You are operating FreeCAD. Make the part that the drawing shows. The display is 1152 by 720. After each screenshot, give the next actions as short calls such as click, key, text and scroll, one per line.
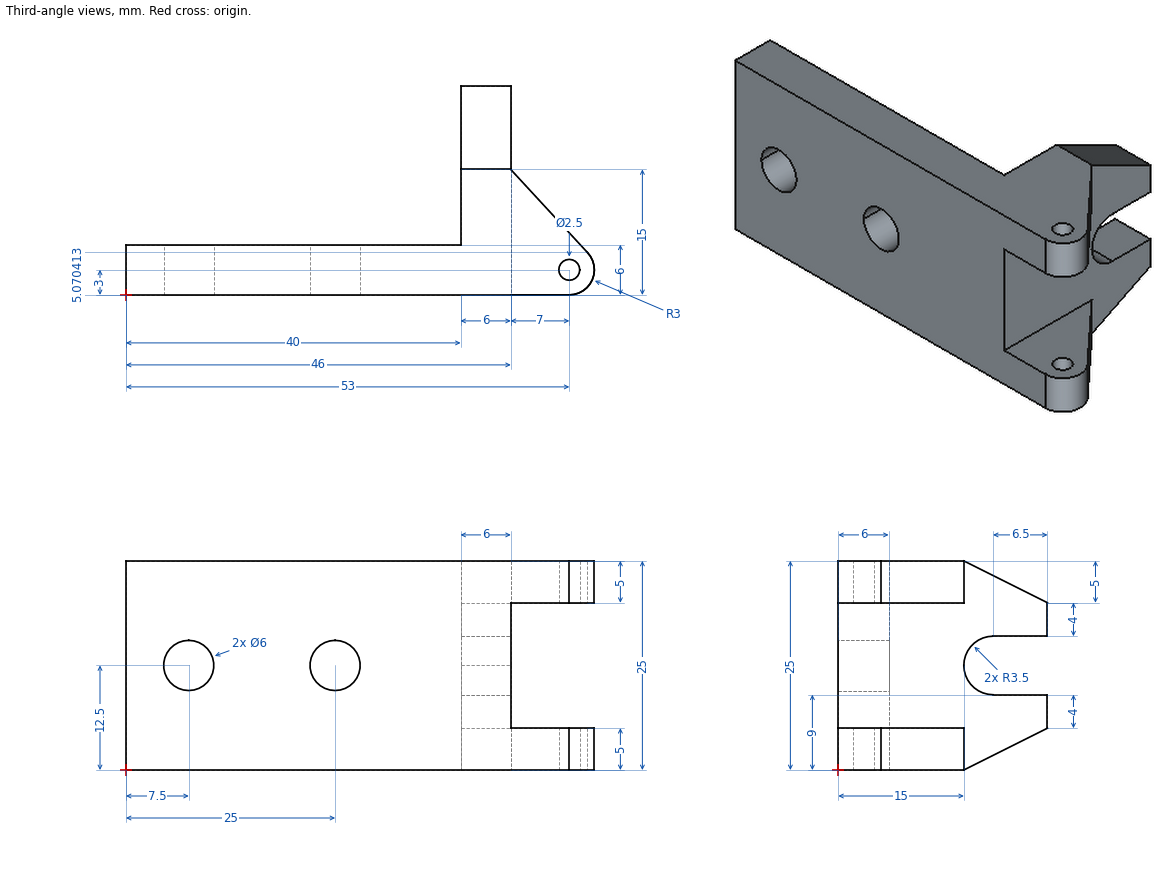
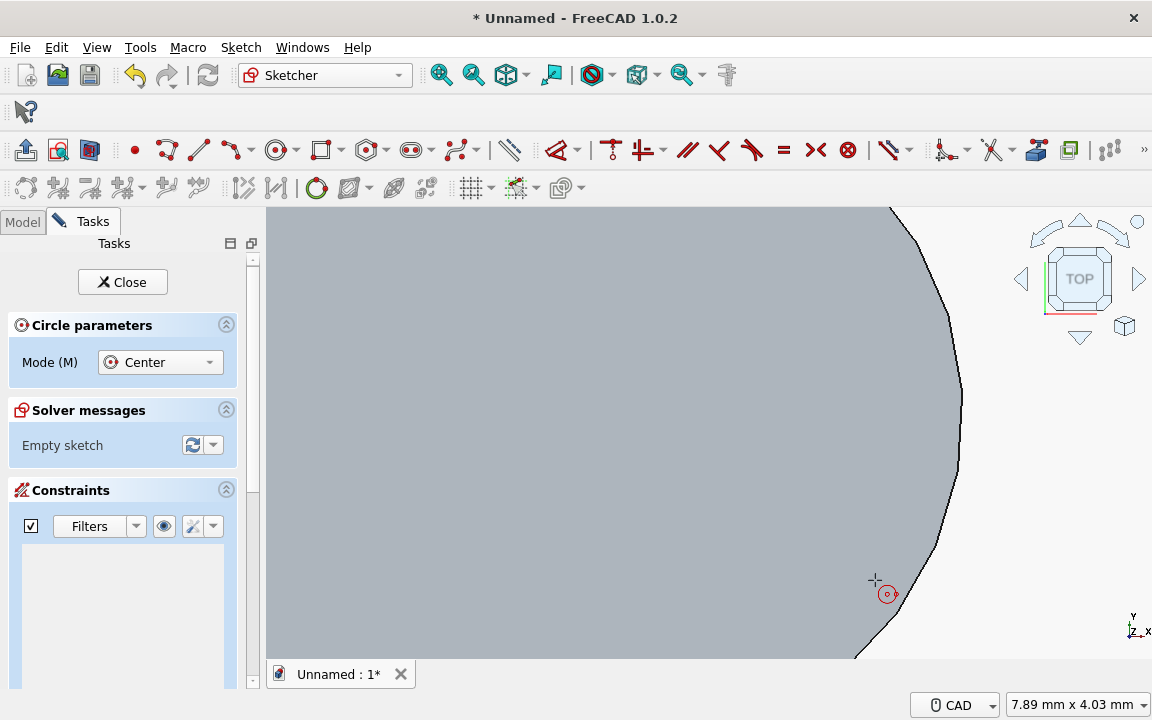
click(626, 413)
click(725, 314)
key(Escape)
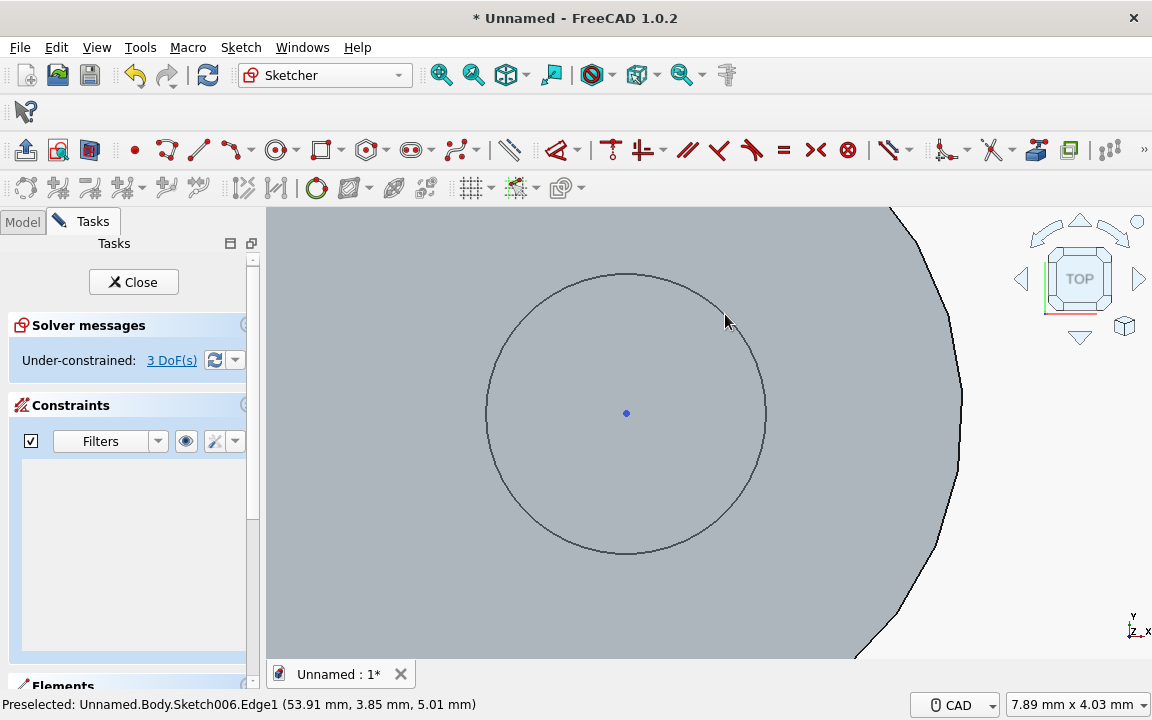
key(d)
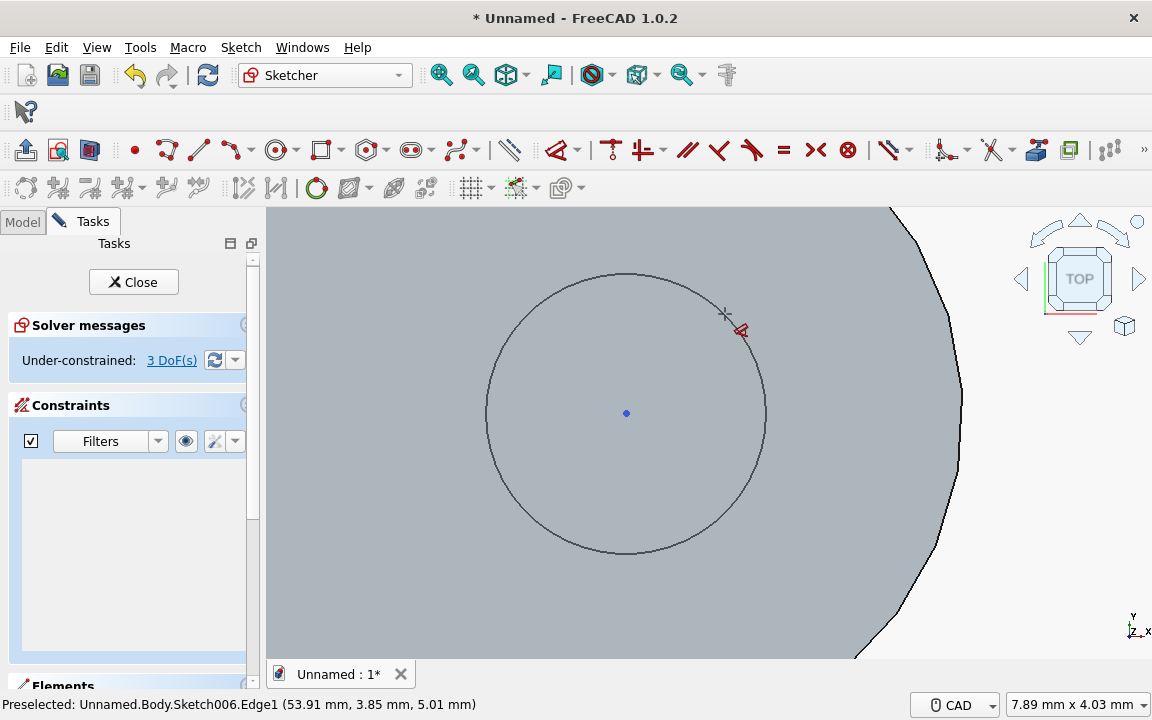
click(725, 315)
click(748, 292)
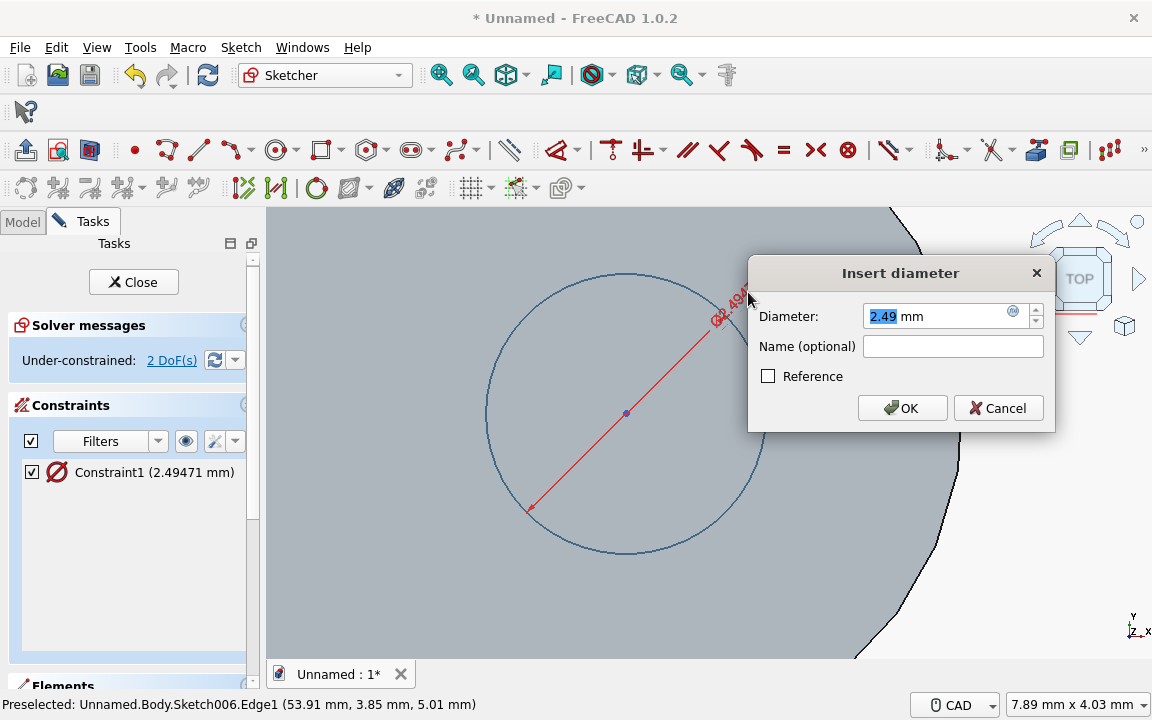
text(2.5)
key(Return)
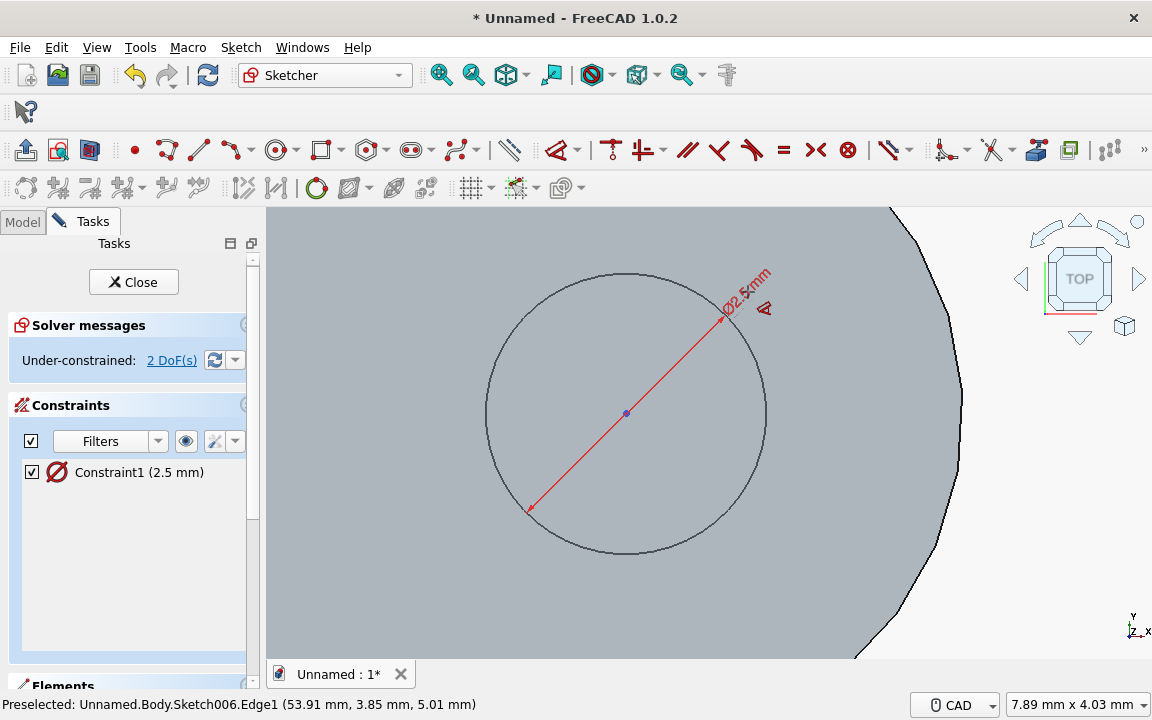
click(626, 414)
click(660, 522)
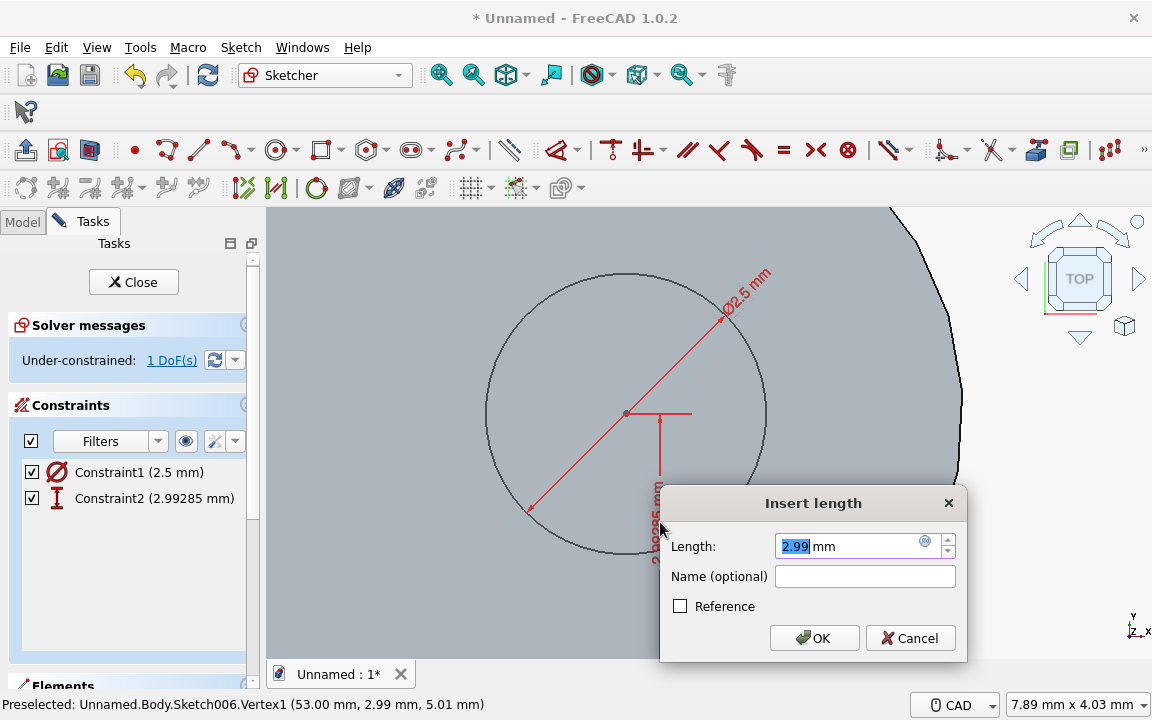
text(3)
key(Return)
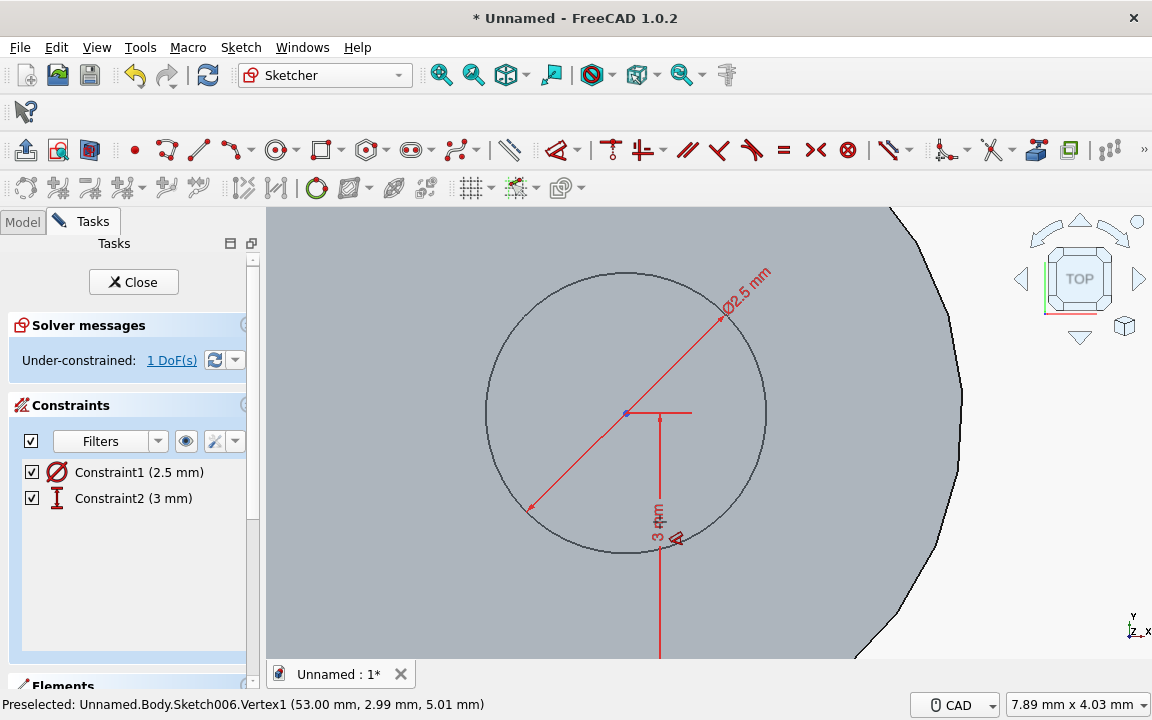
click(626, 413)
click(460, 379)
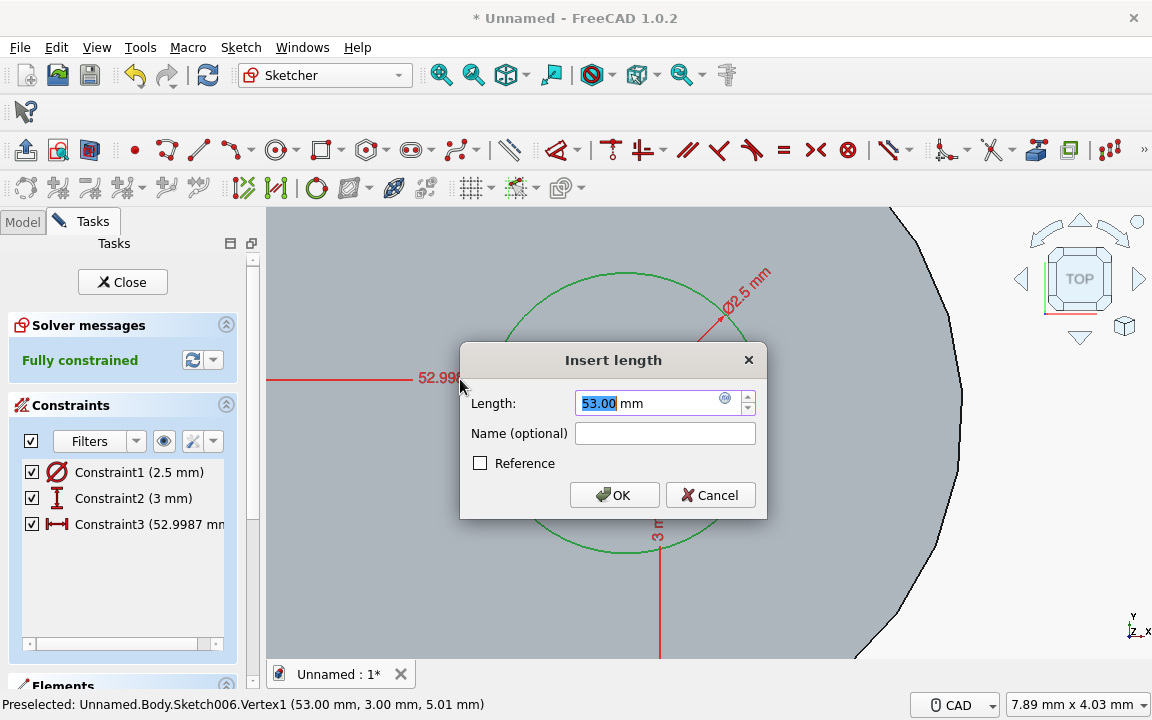
text(53)
key(Return)
key(Escape)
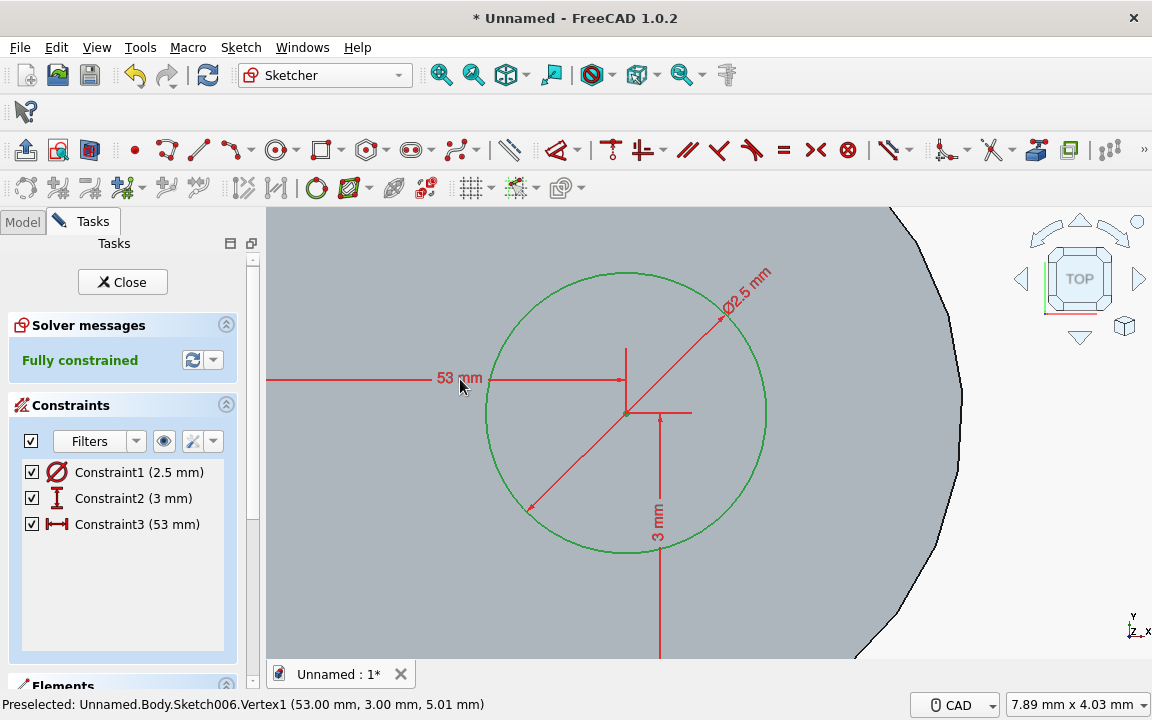
click(123, 282)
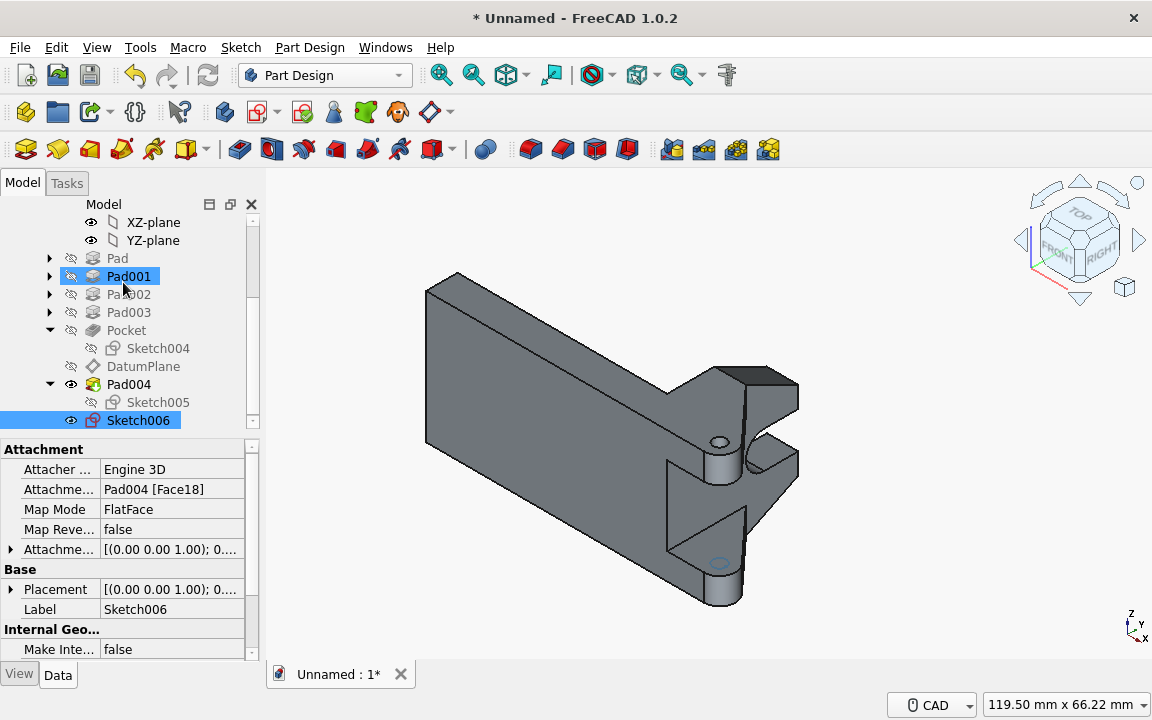
click(240, 150)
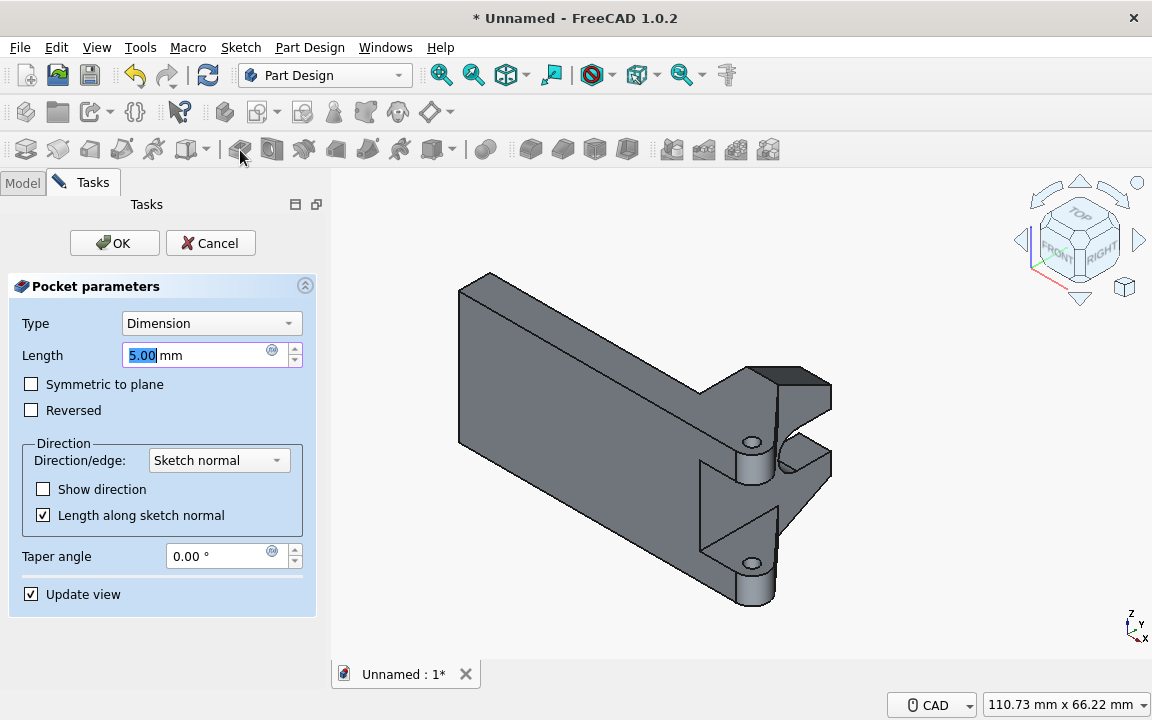
text(5)
key(Tab)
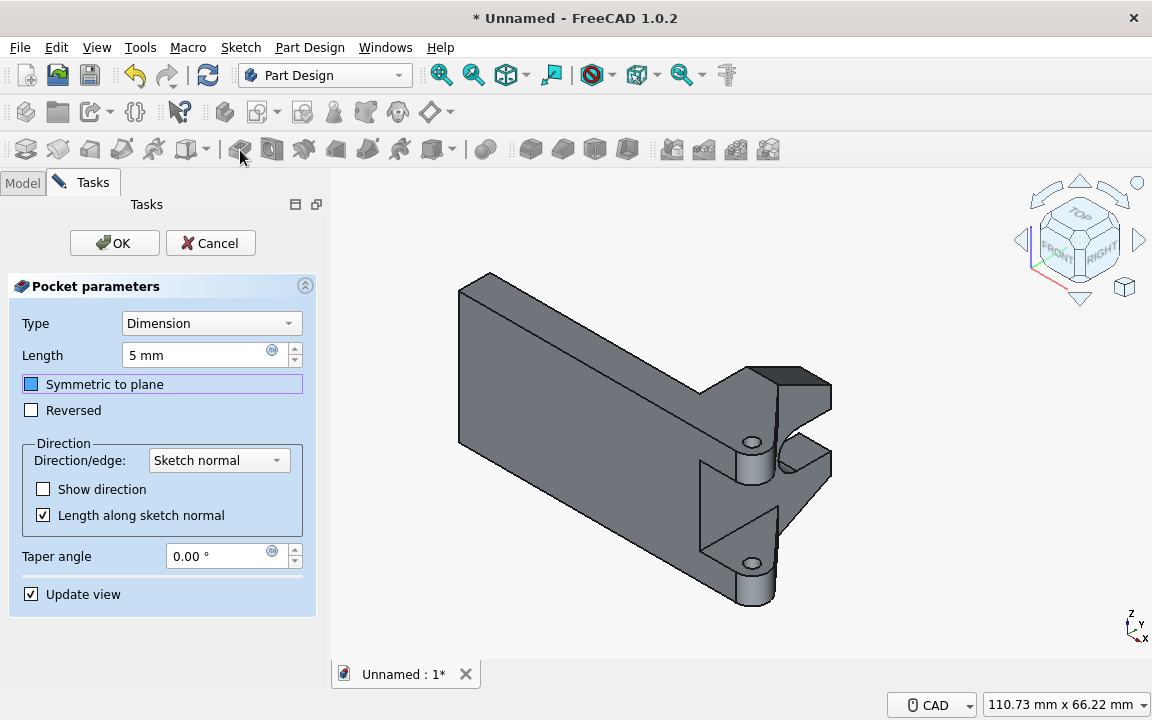
click(115, 243)